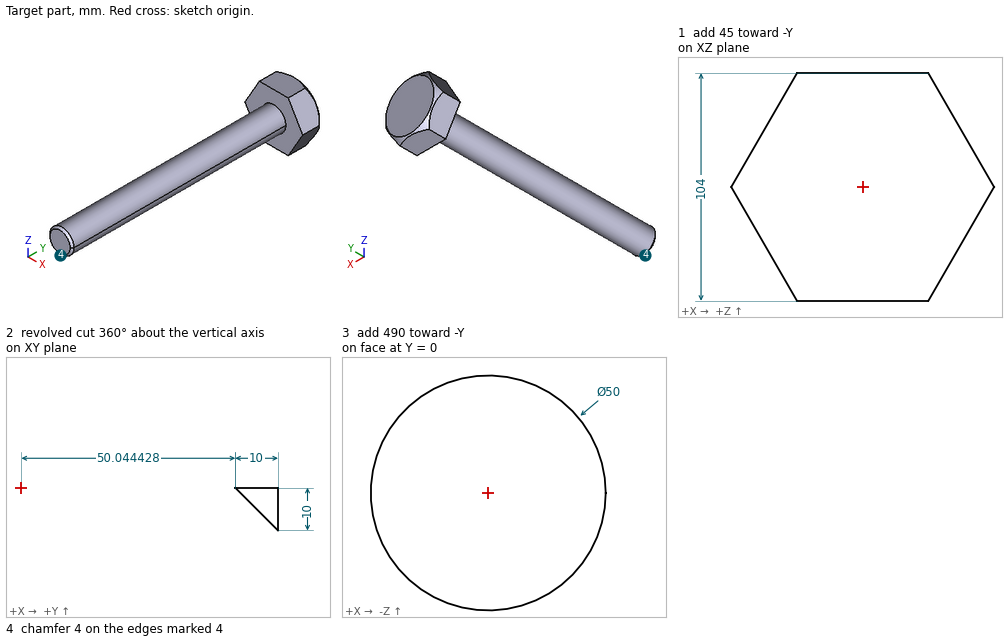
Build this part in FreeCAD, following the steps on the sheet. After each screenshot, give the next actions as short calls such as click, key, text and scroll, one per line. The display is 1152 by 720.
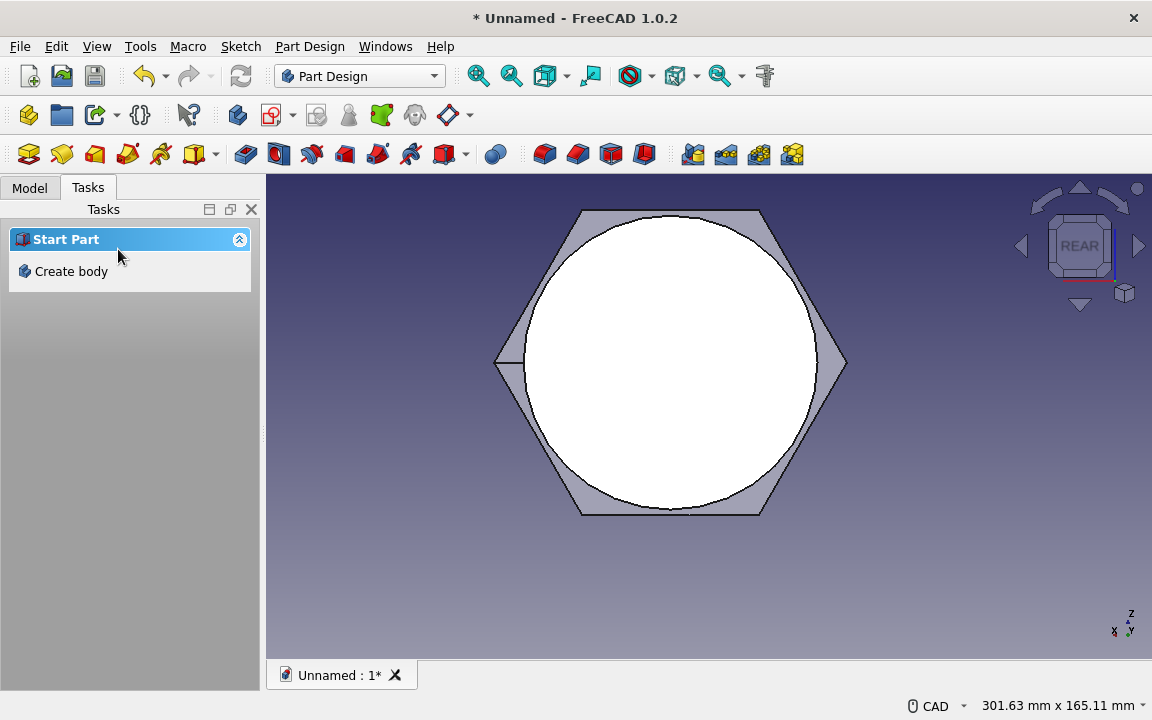
key(0)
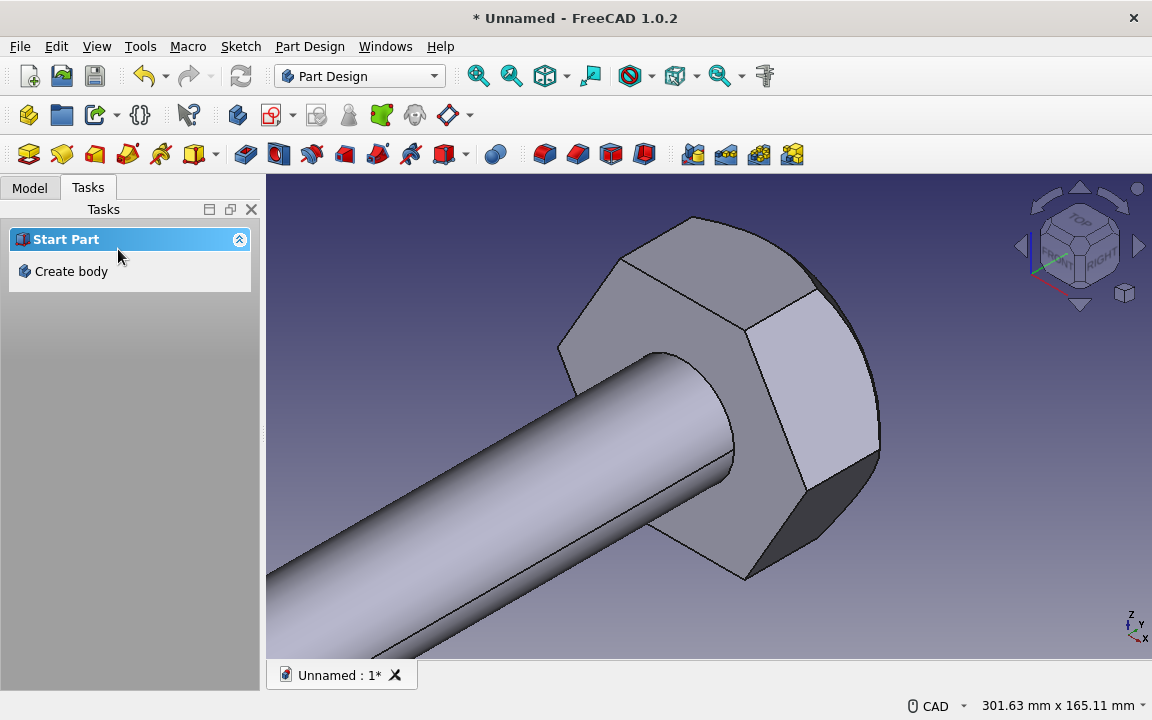
key(v)
key(f)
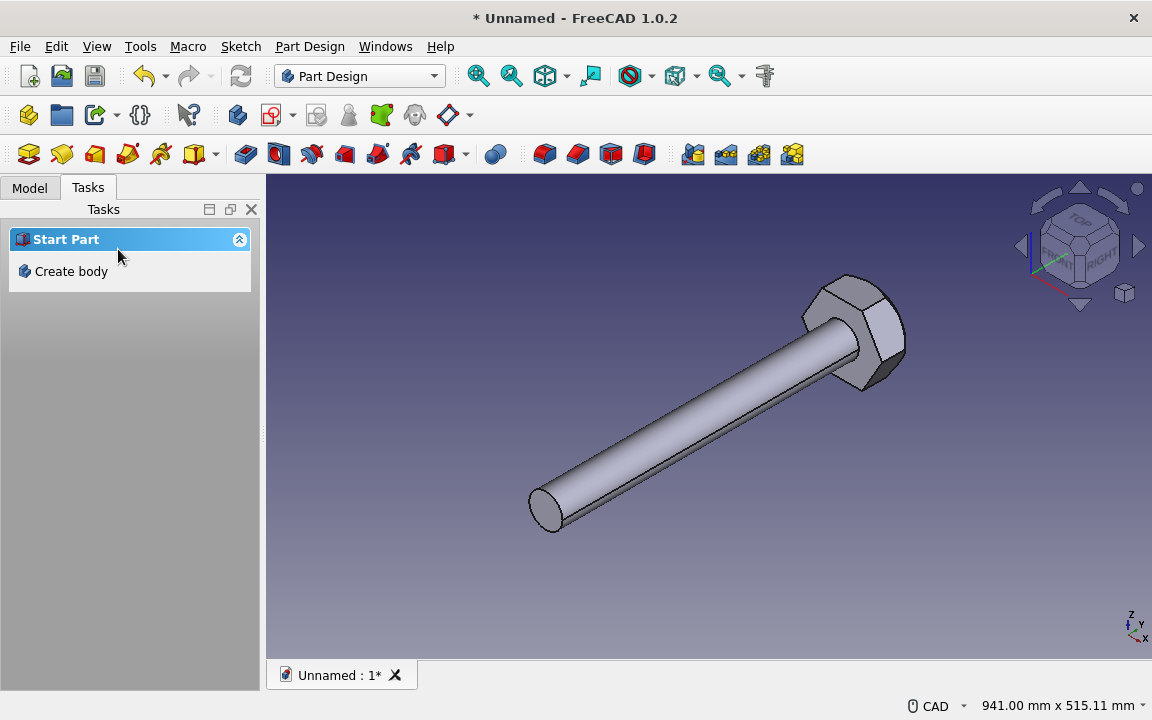
click(532, 491)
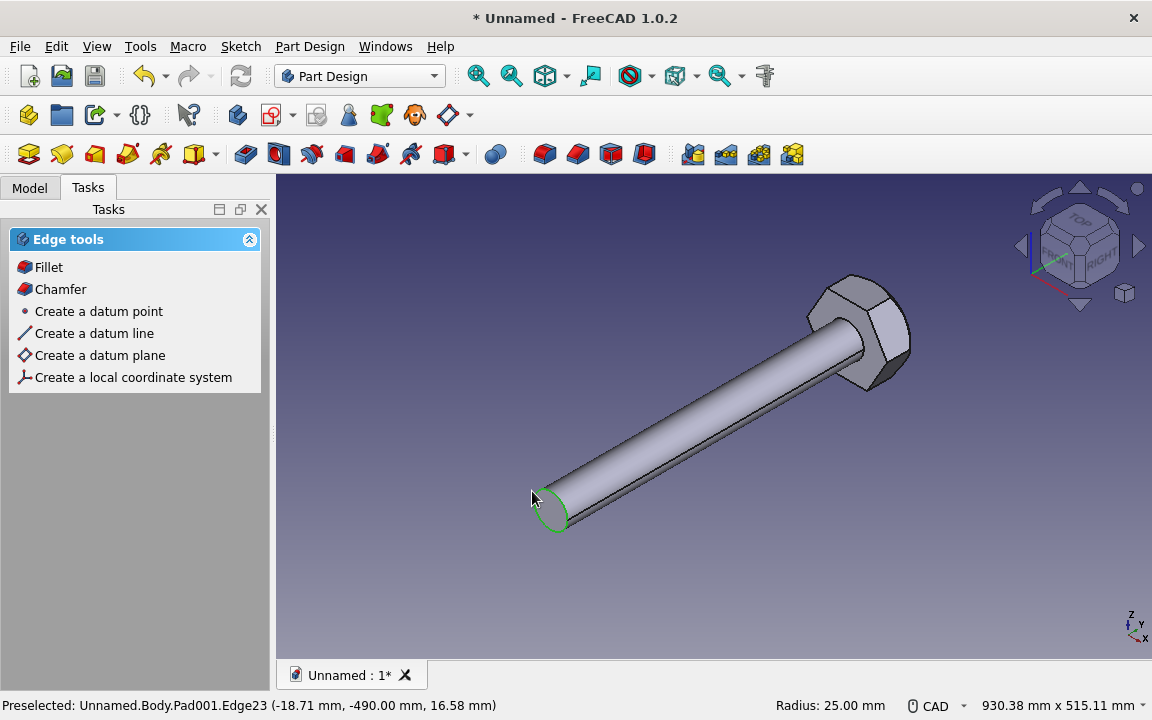
click(578, 154)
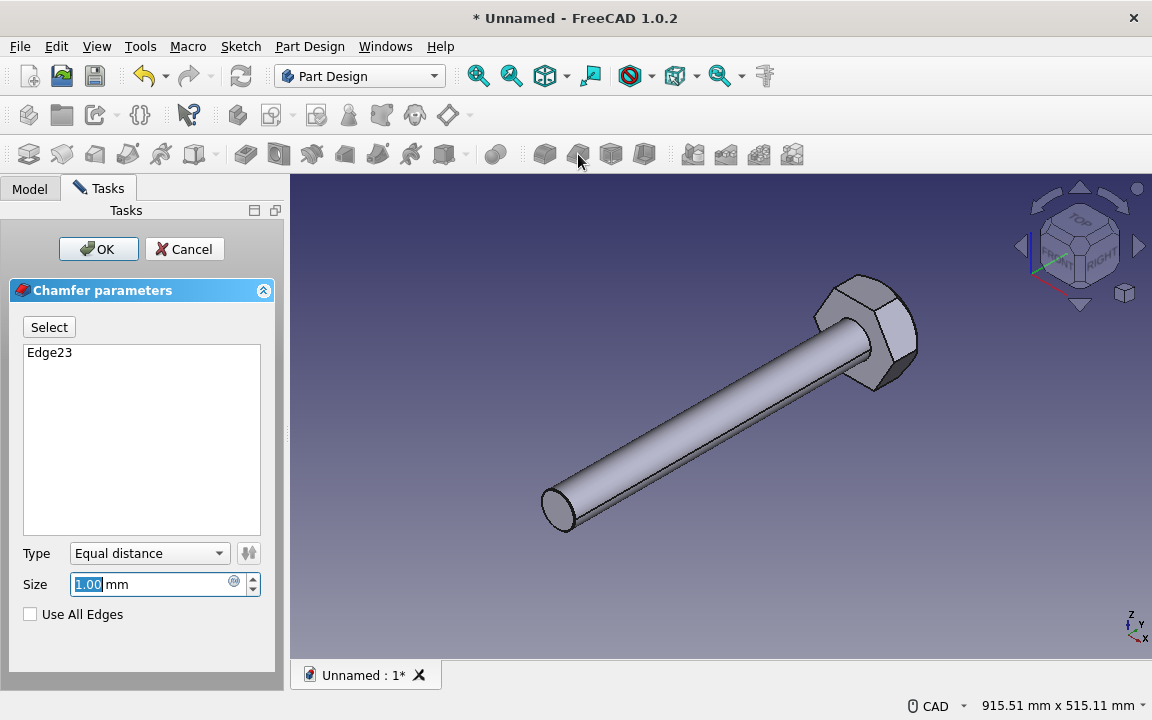
text(4)
key(Tab)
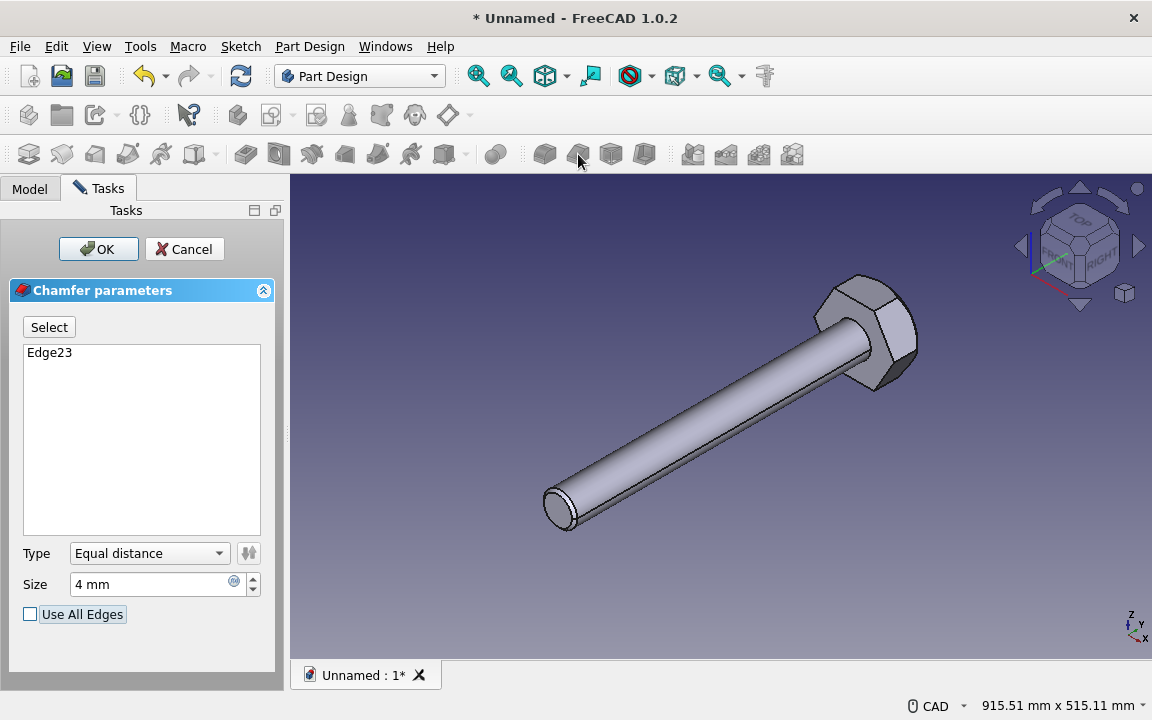
click(99, 249)